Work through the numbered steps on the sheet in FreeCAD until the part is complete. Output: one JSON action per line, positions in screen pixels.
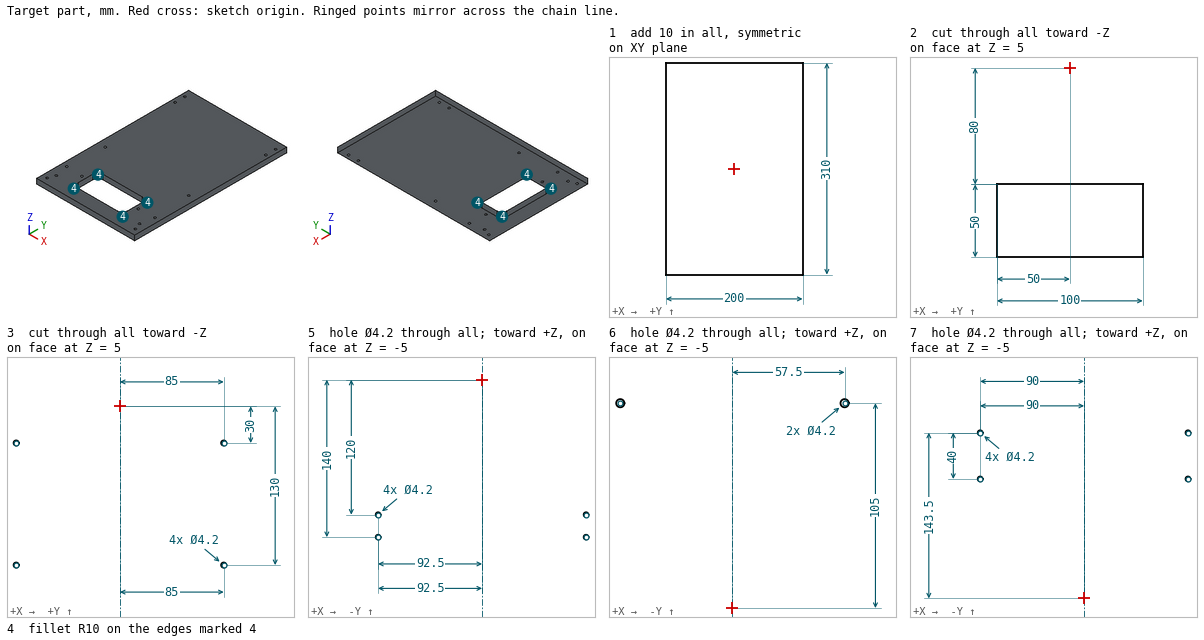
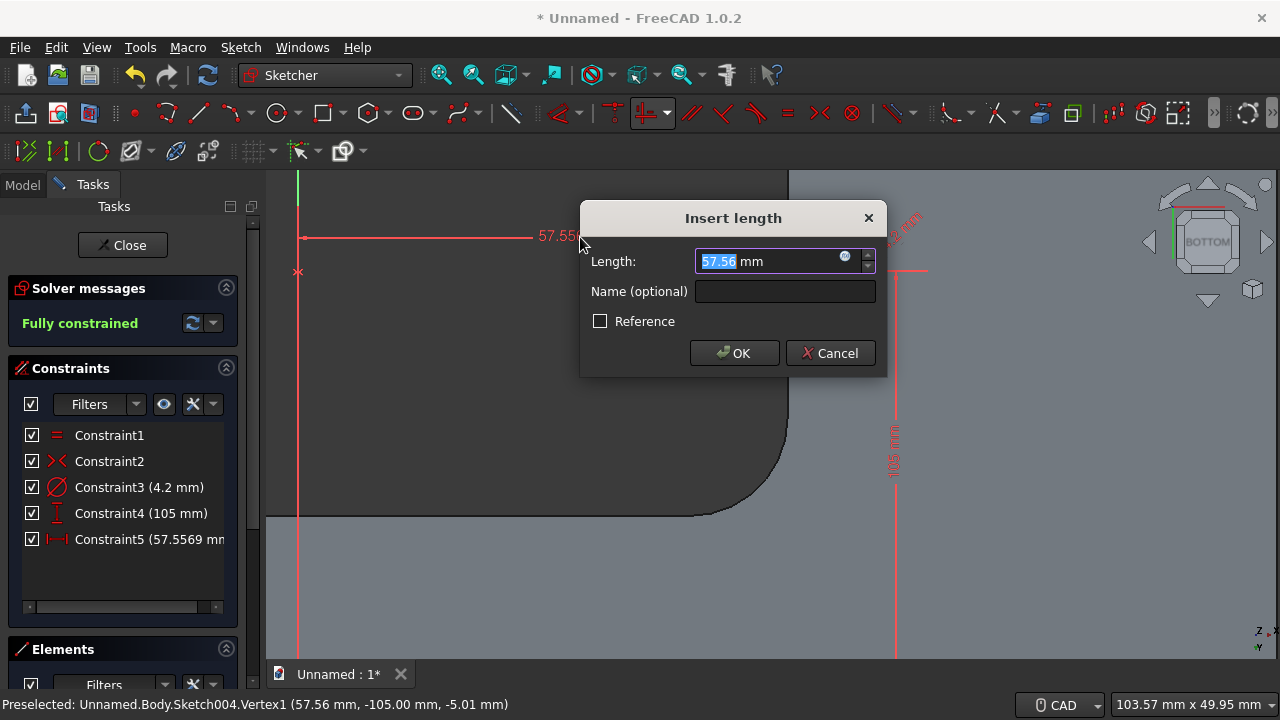
{"action": "type", "text": "57.5"}
{"action": "key", "text": "Return"}
{"action": "key", "text": "Escape"}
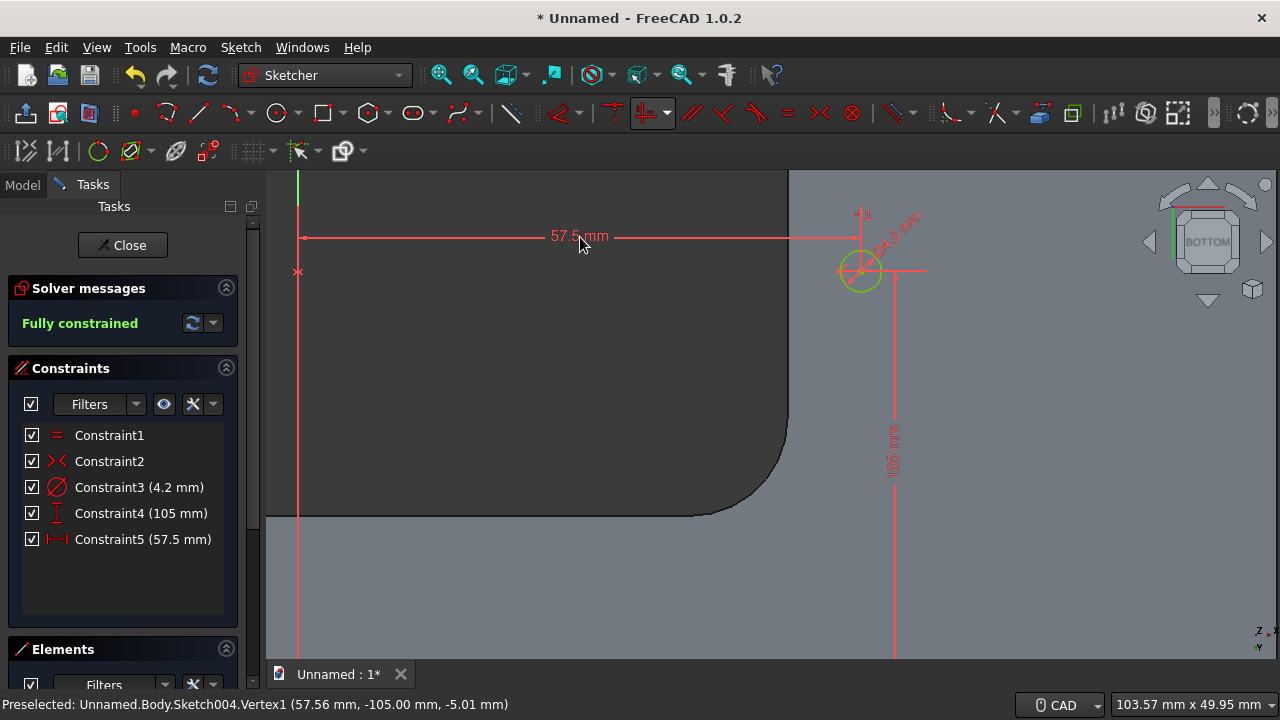
{"action": "left_click", "coordinate": [123, 245]}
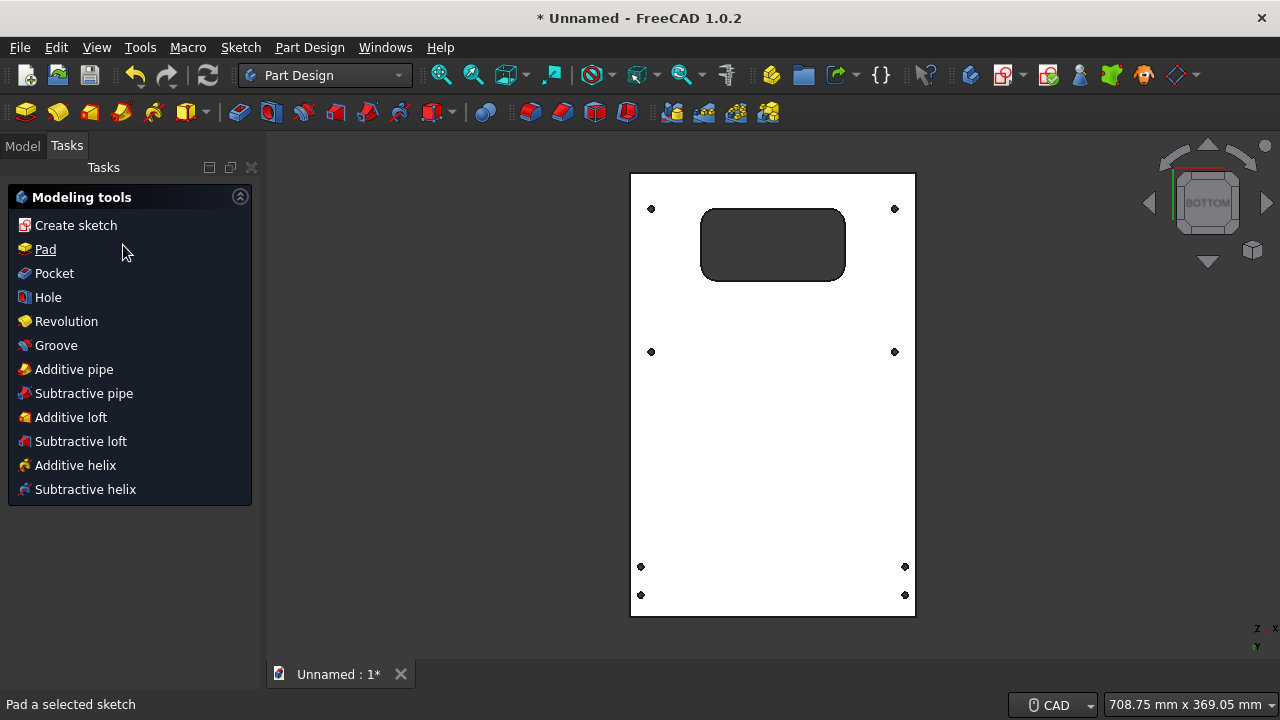
{"action": "left_click", "coordinate": [272, 112]}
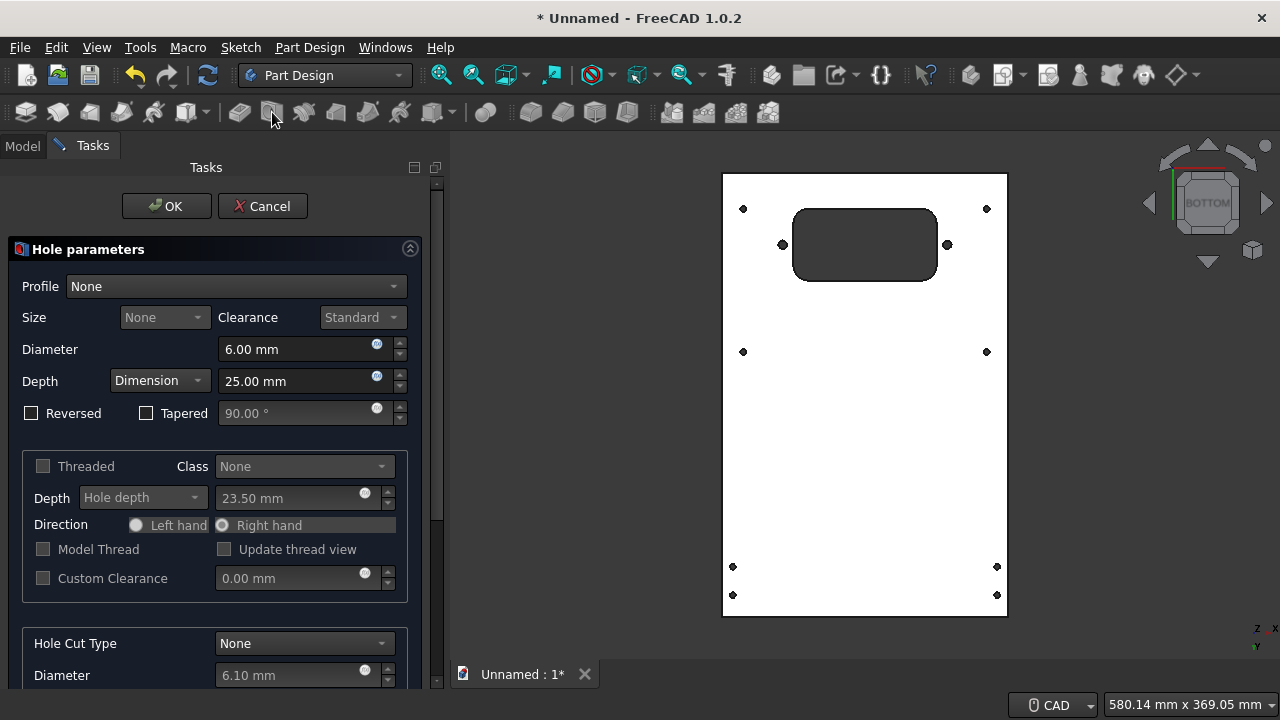
{"action": "triple_click", "coordinate": [305, 349]}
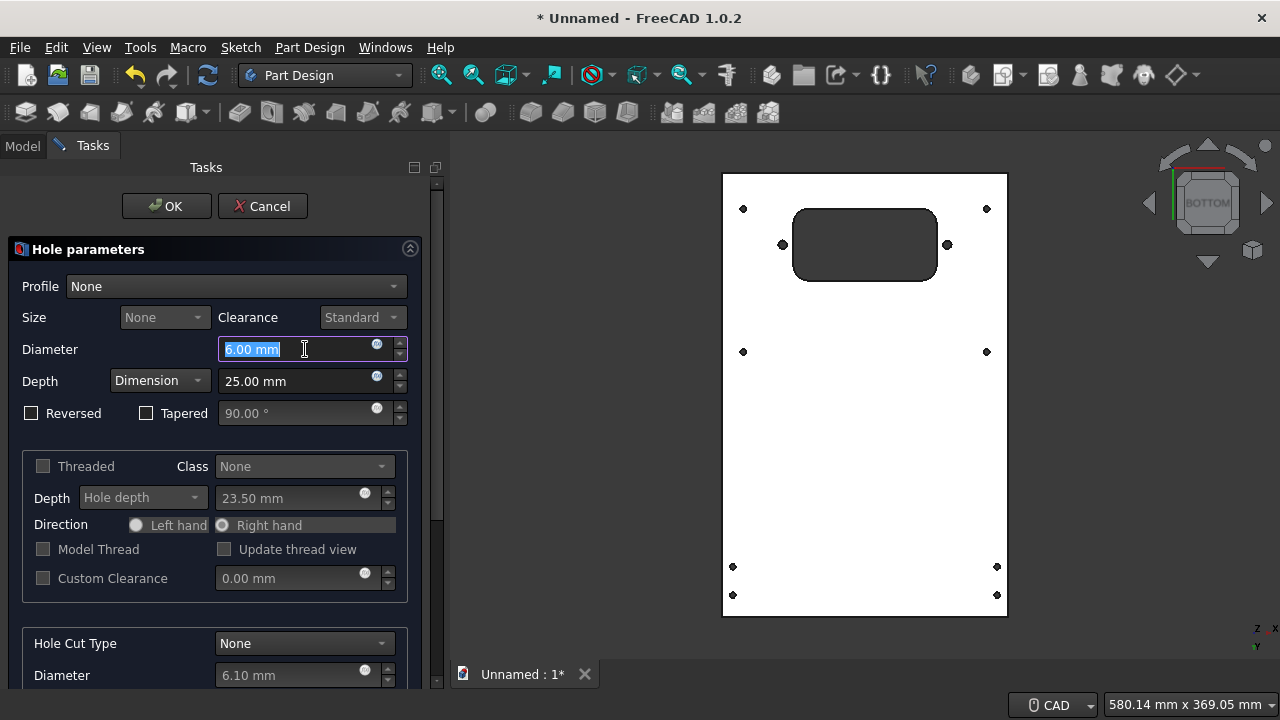
{"action": "type", "text": "4.2"}
{"action": "key", "text": "Tab"}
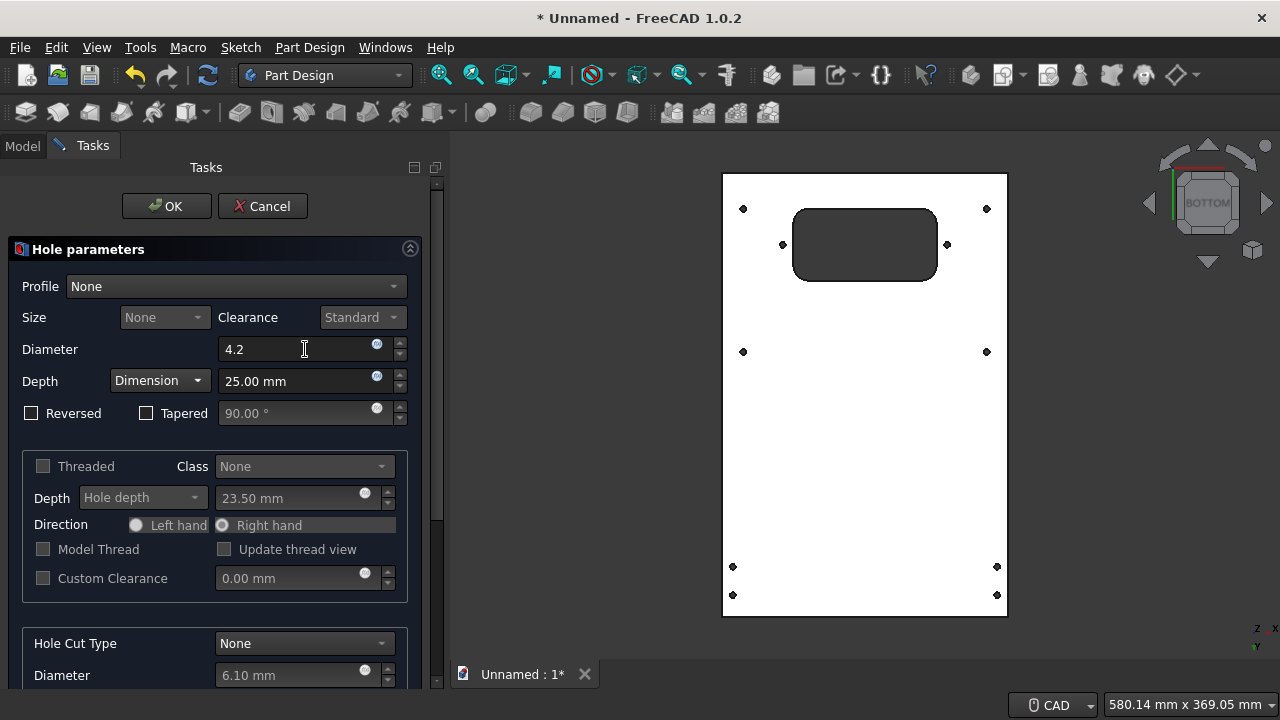
{"action": "left_click", "coordinate": [161, 380]}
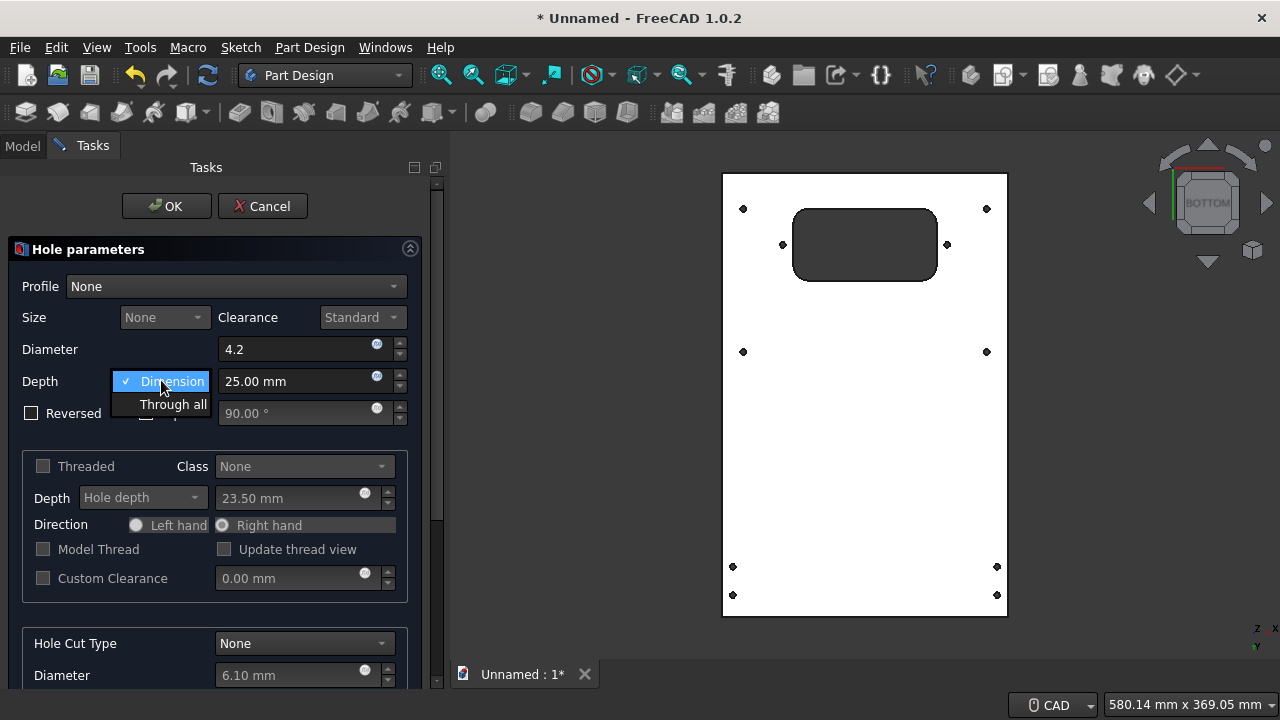
{"action": "left_click", "coordinate": [160, 404]}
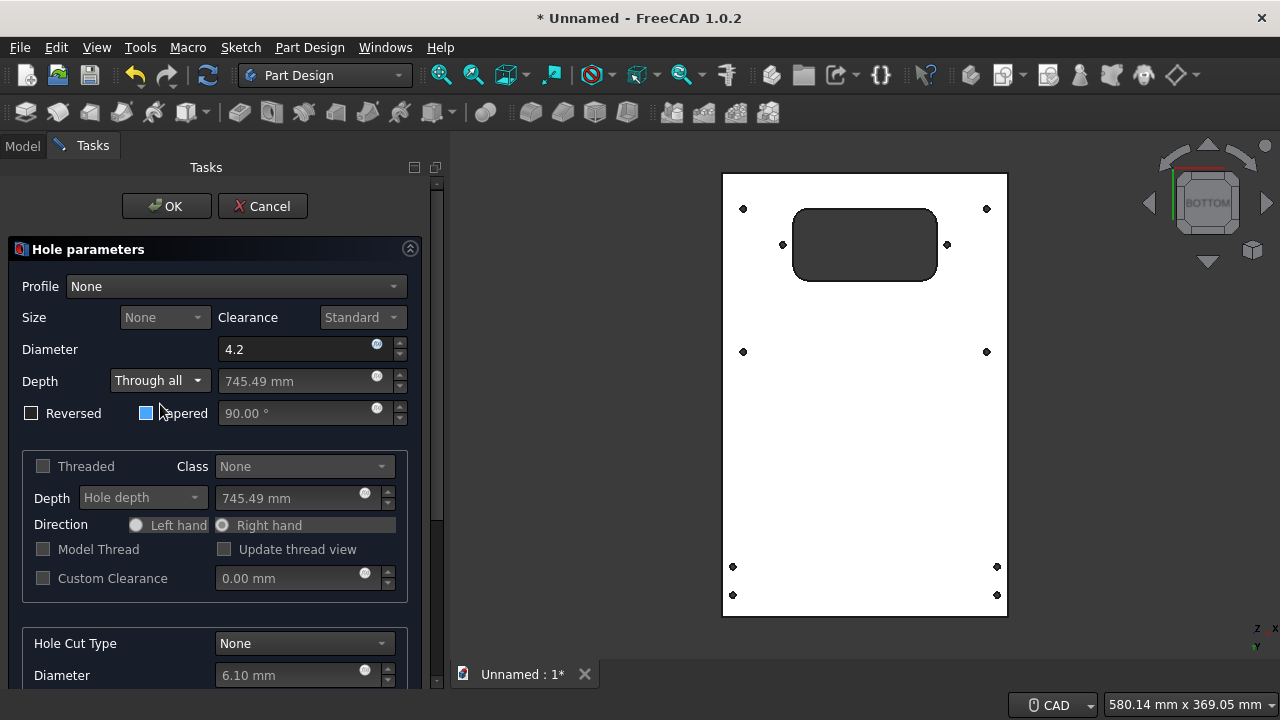
{"action": "left_click", "coordinate": [167, 206]}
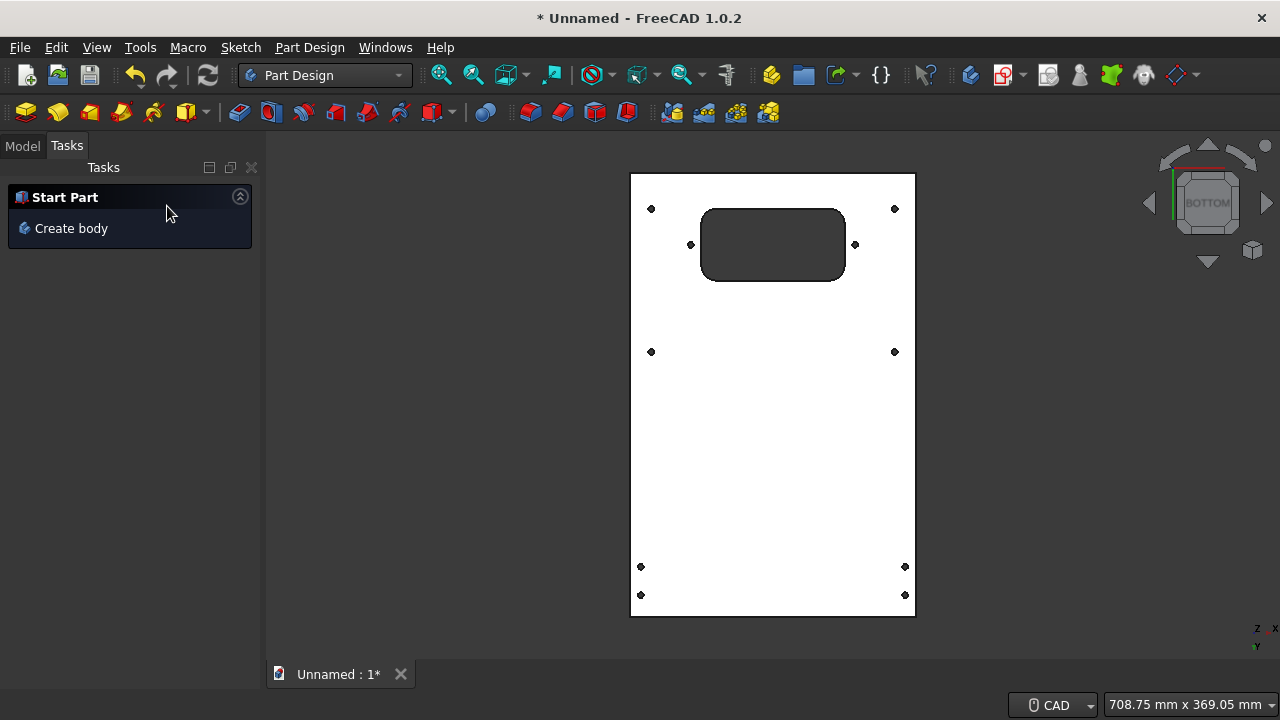
{"action": "left_click", "coordinate": [773, 457]}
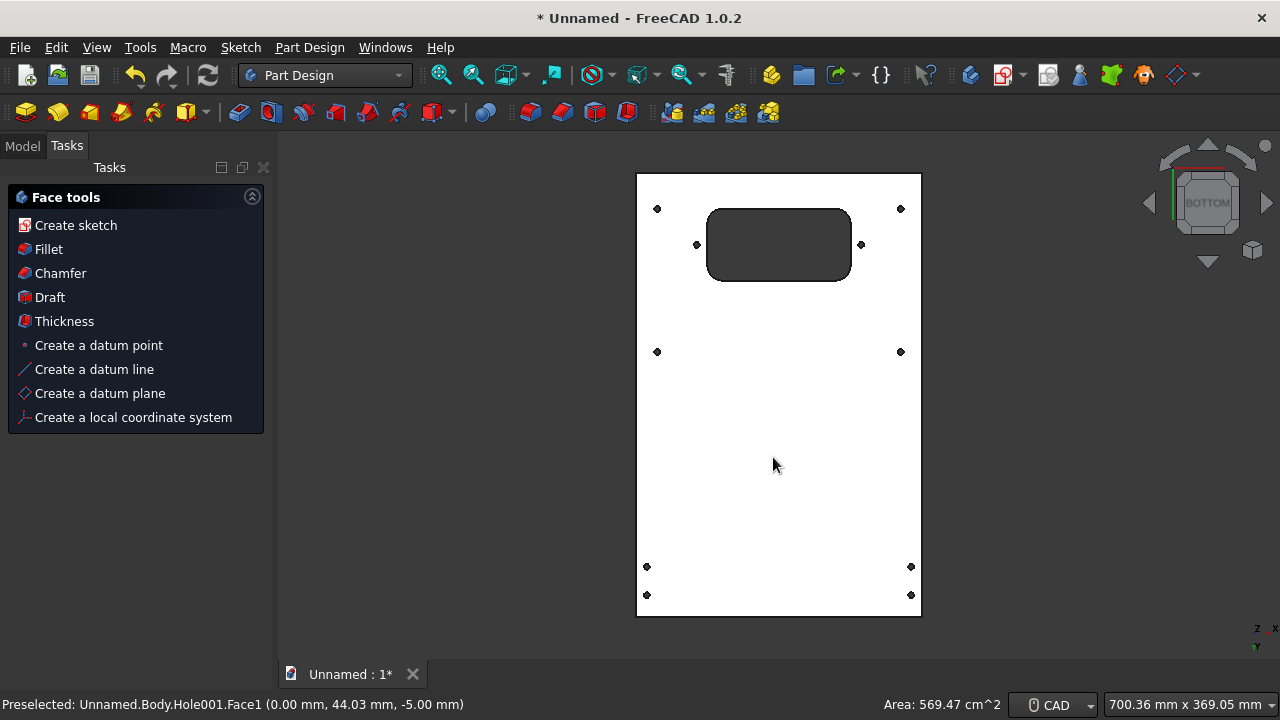
{"action": "left_click", "coordinate": [1004, 76]}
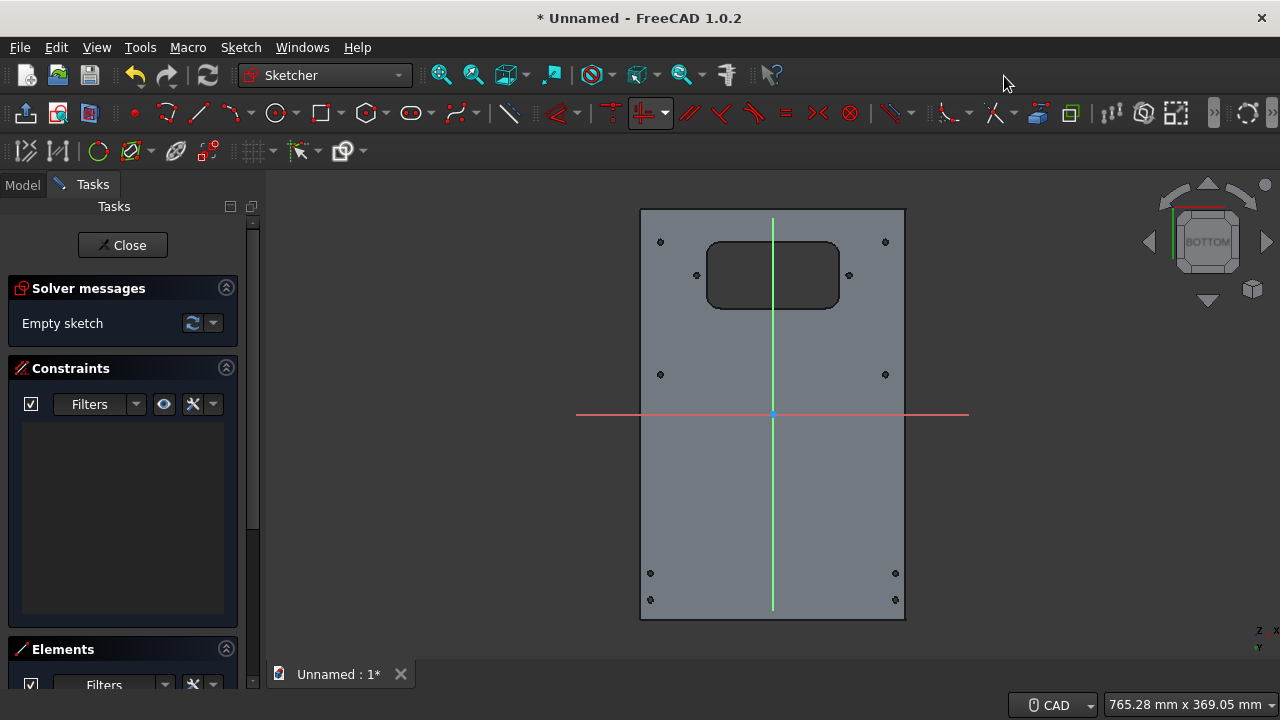
{"action": "scroll", "coordinate": [912, 198], "scroll_direction": "up", "scroll_amount": 2}